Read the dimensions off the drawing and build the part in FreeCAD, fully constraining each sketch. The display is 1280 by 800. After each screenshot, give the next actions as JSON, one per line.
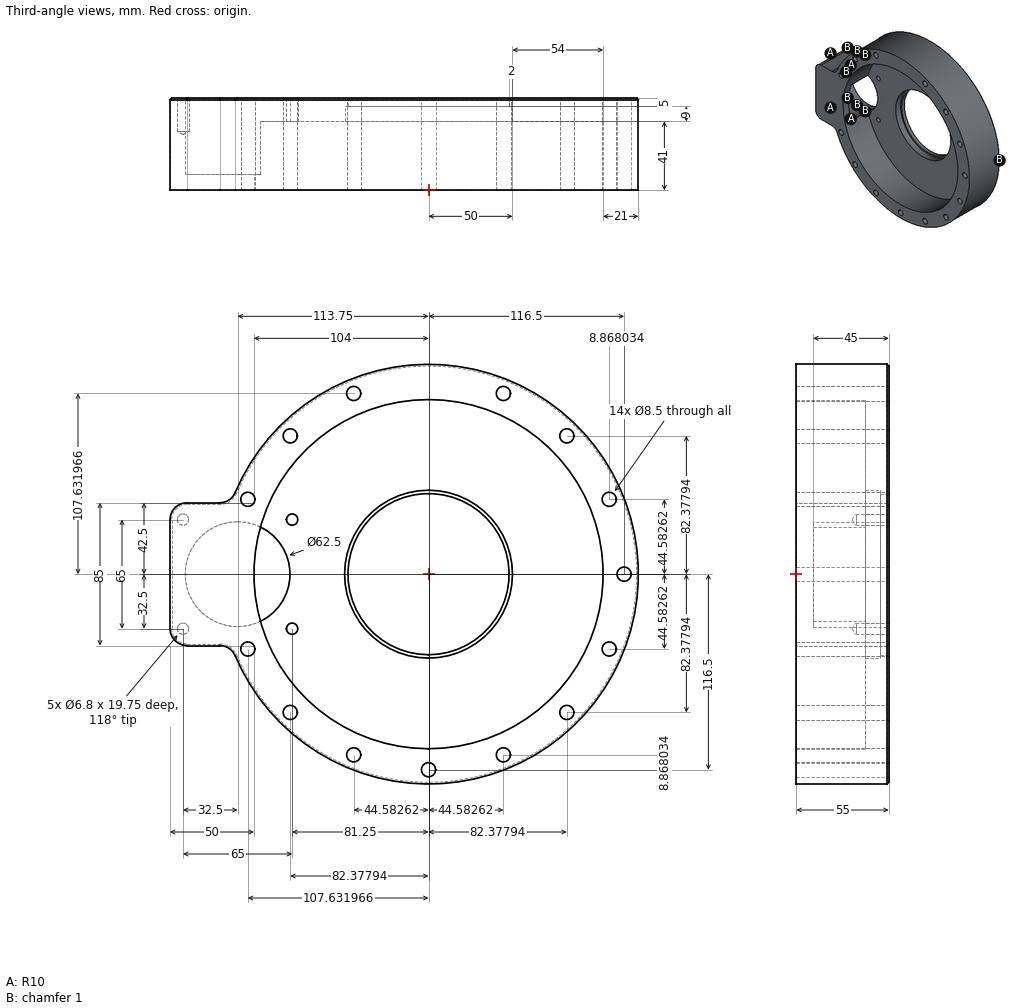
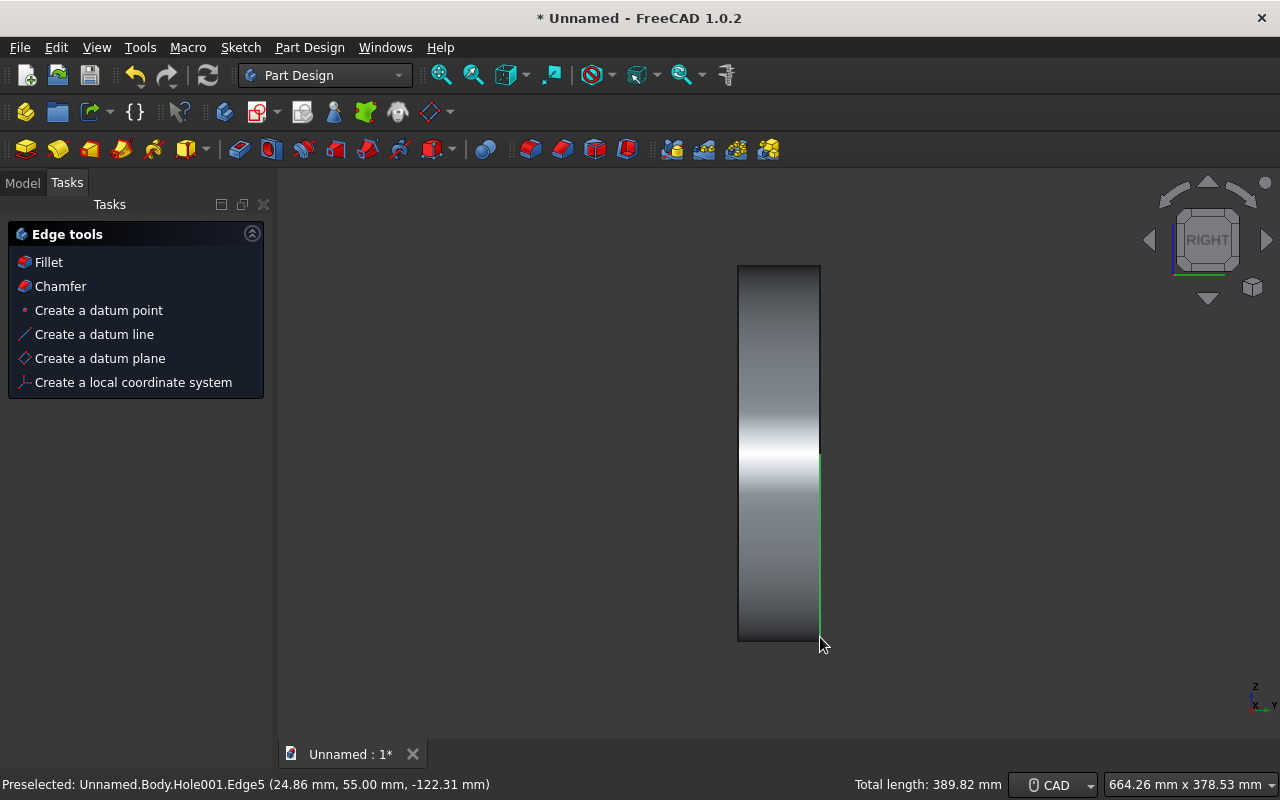
{"action": "key", "text": "5"}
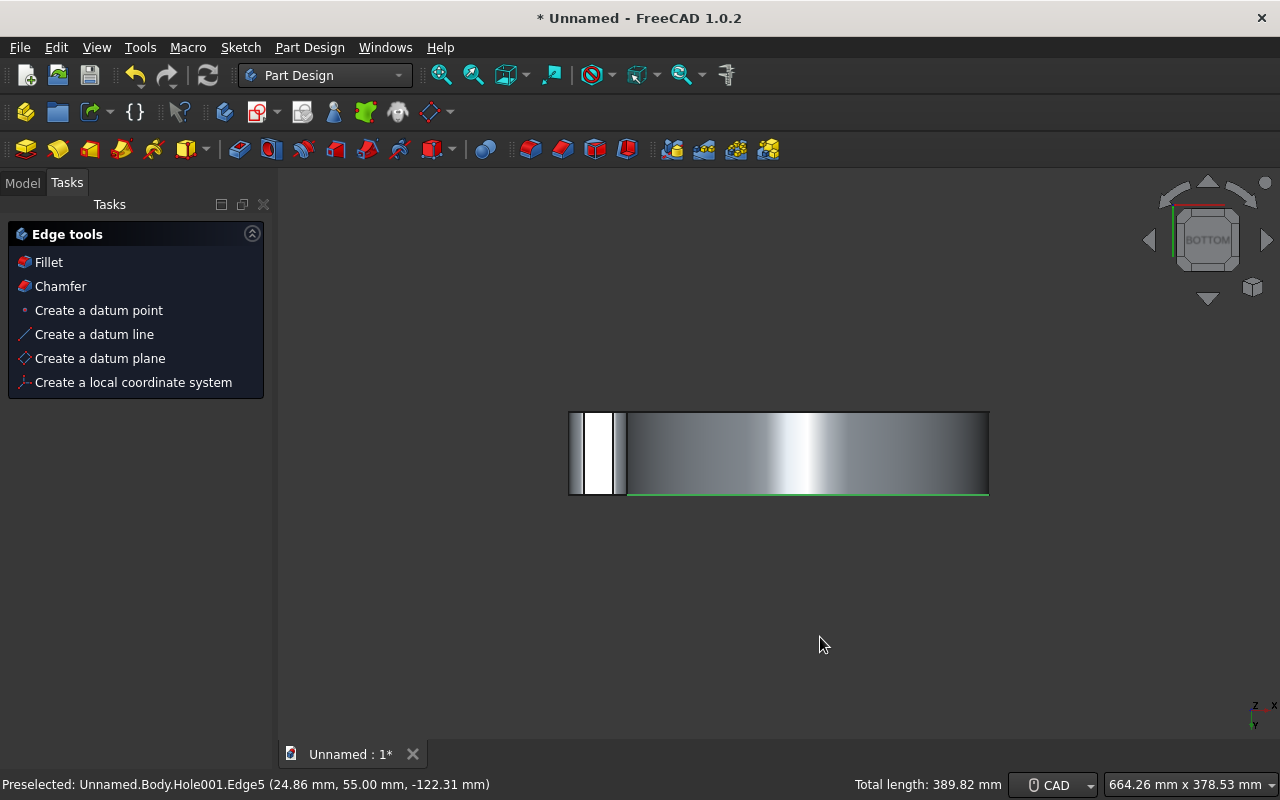
{"action": "left_click", "coordinate": [442, 76]}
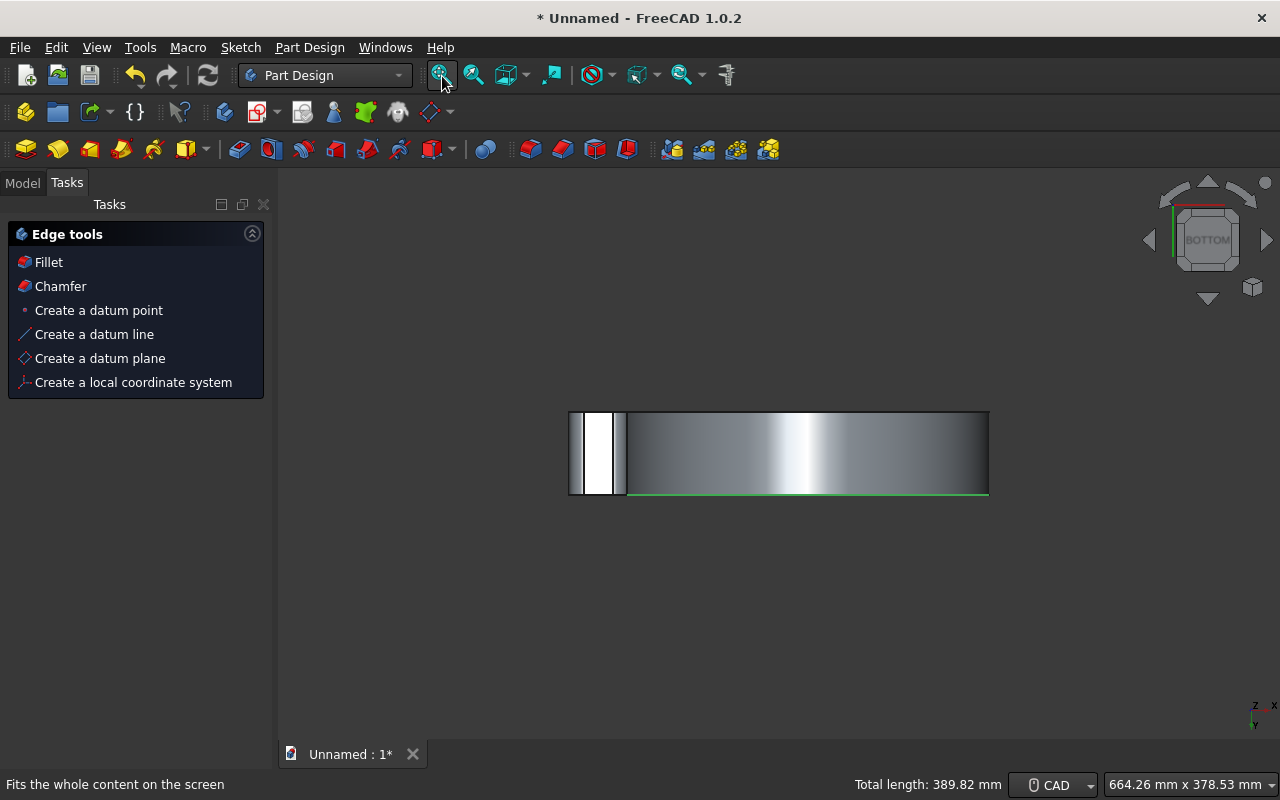
{"action": "left_click", "coordinate": [598, 494], "text": "ctrl"}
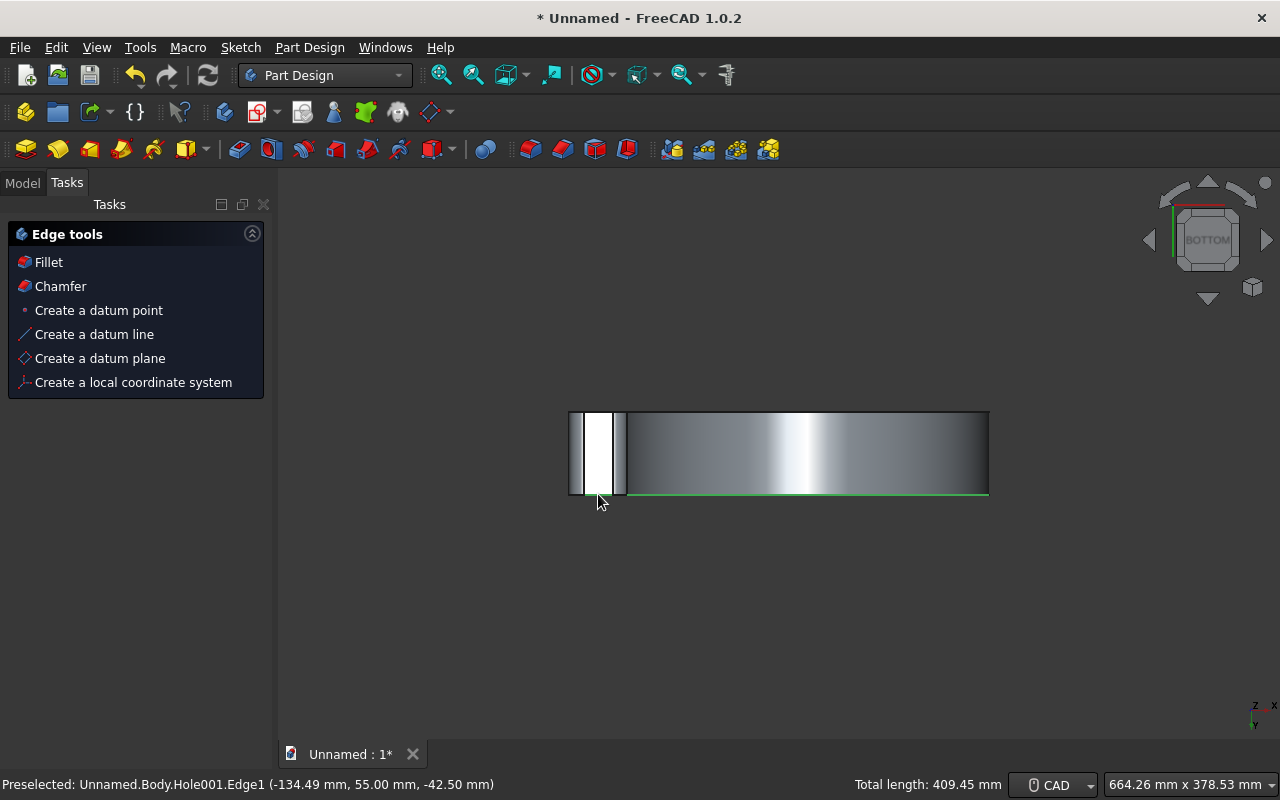
{"action": "left_click", "coordinate": [573, 494], "text": "ctrl"}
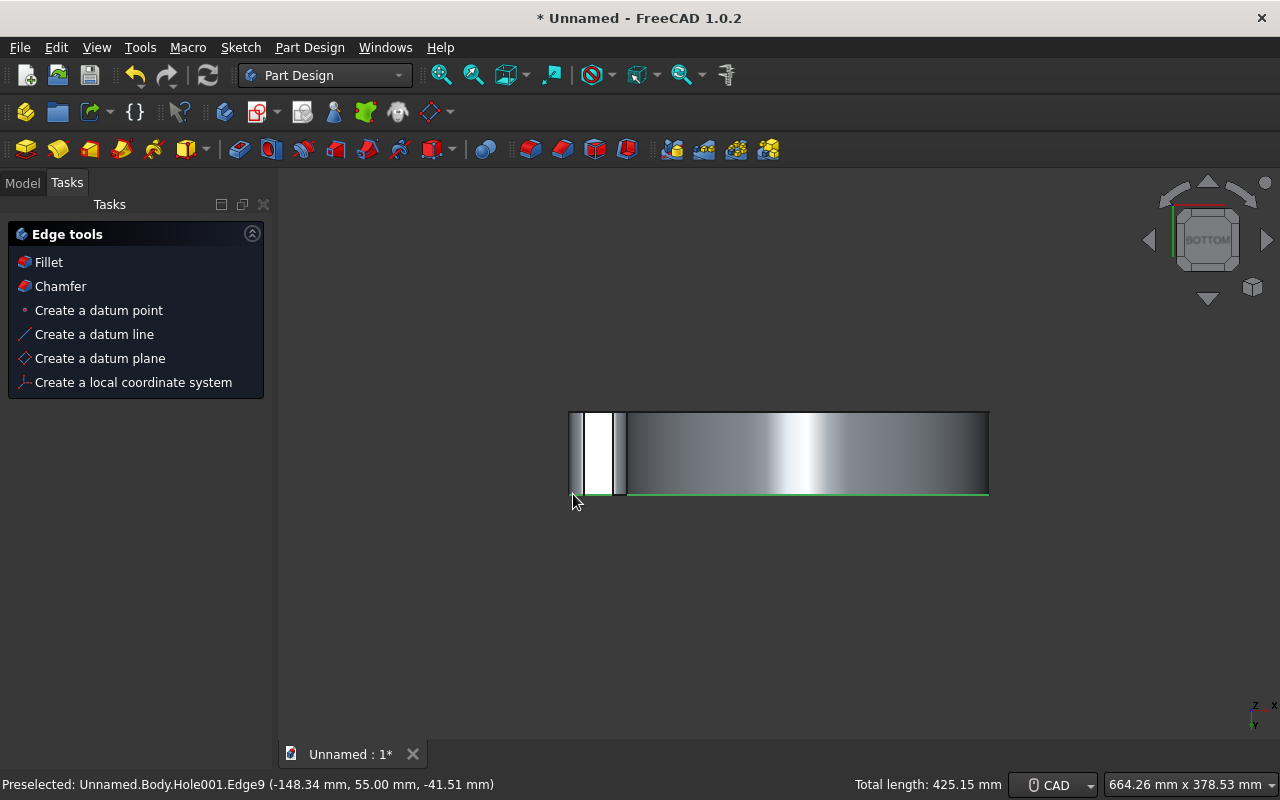
{"action": "left_click", "coordinate": [620, 494], "text": "ctrl"}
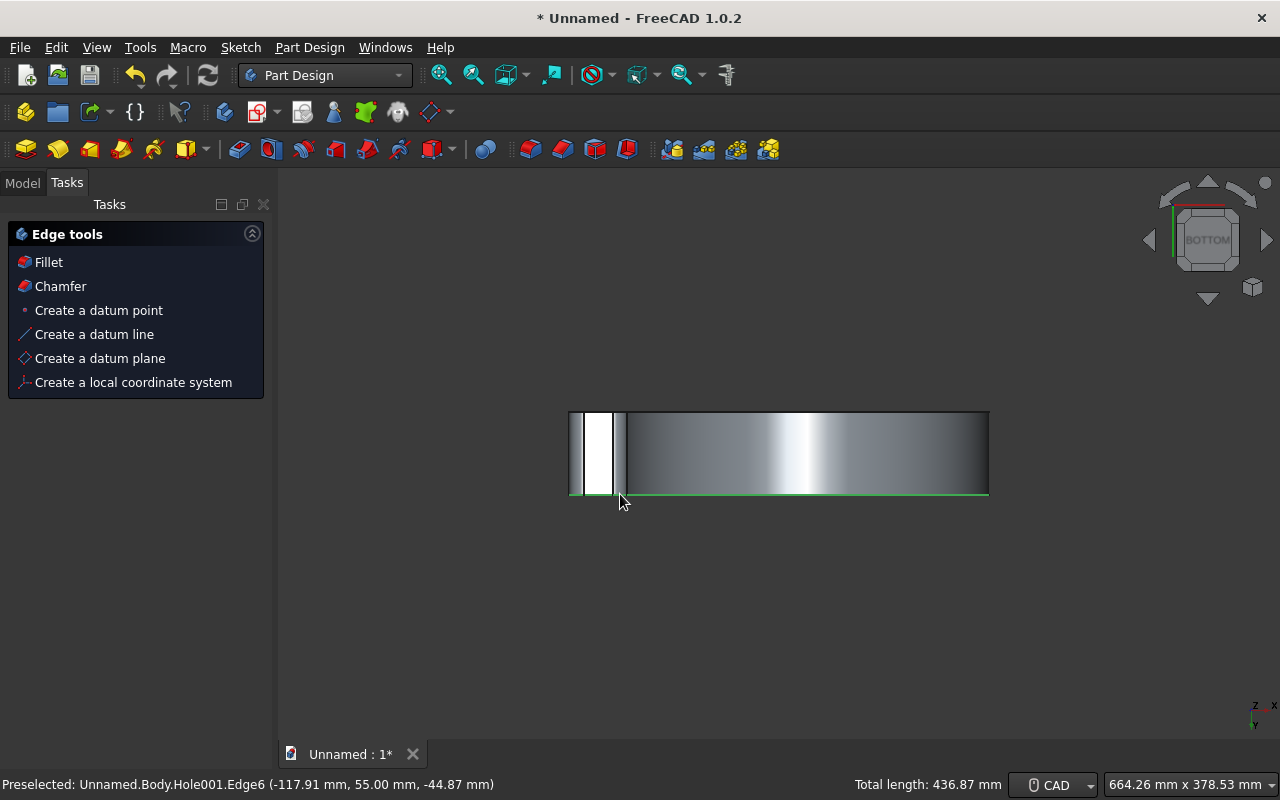
{"action": "key", "text": "4"}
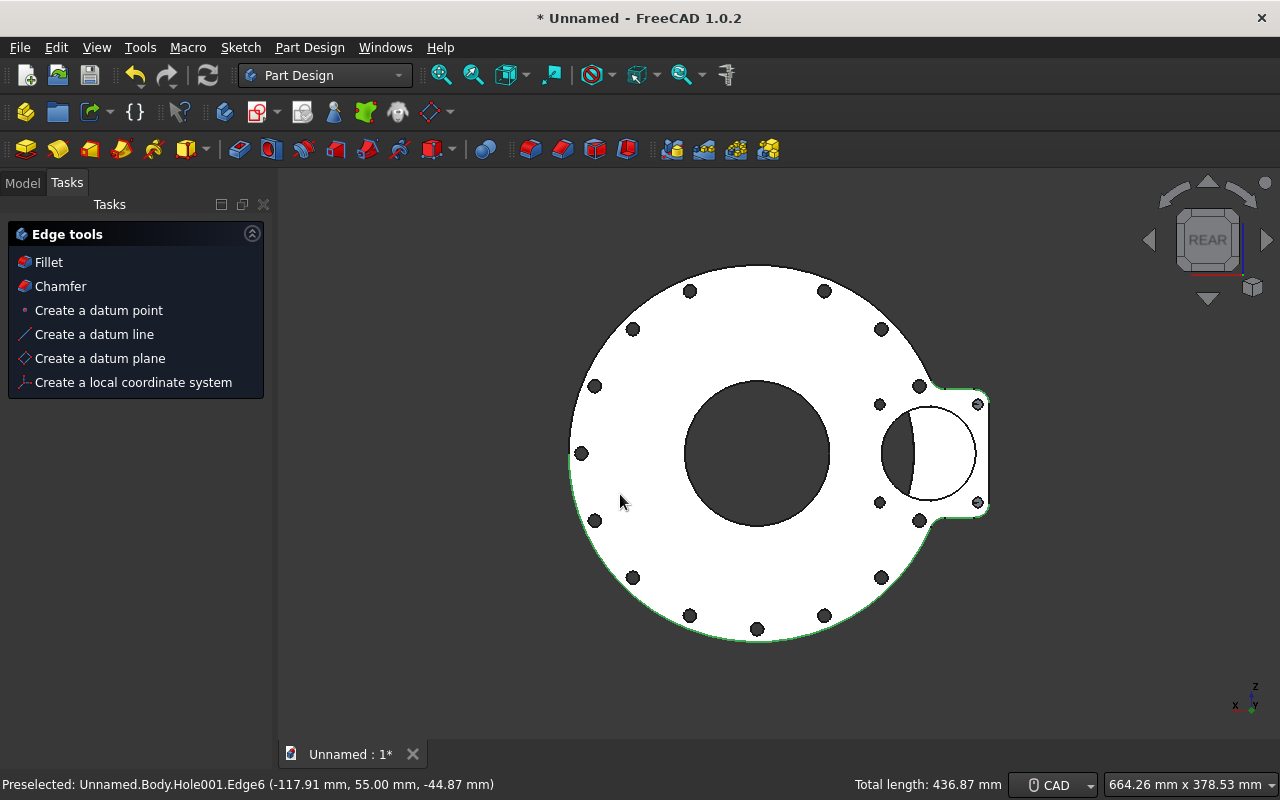
{"action": "left_click", "coordinate": [989, 452], "text": "ctrl"}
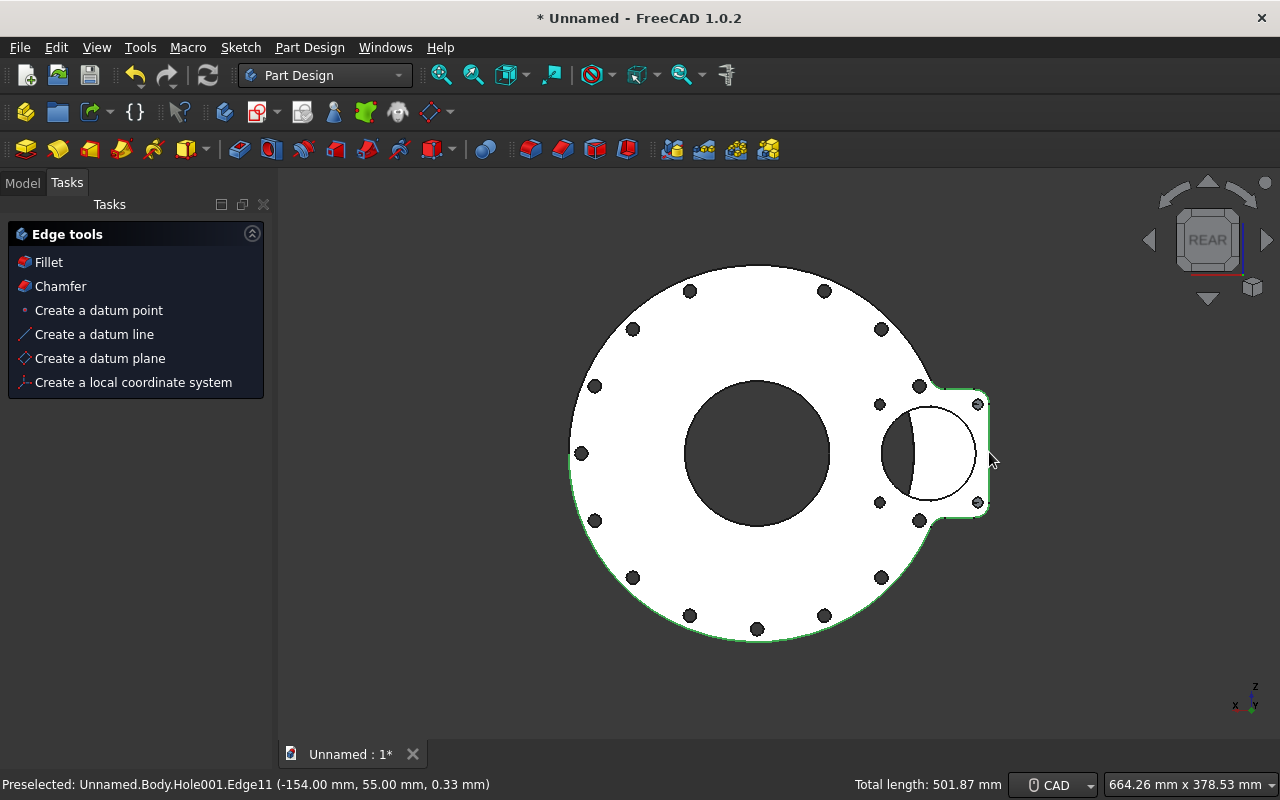
{"action": "left_click", "coordinate": [564, 150]}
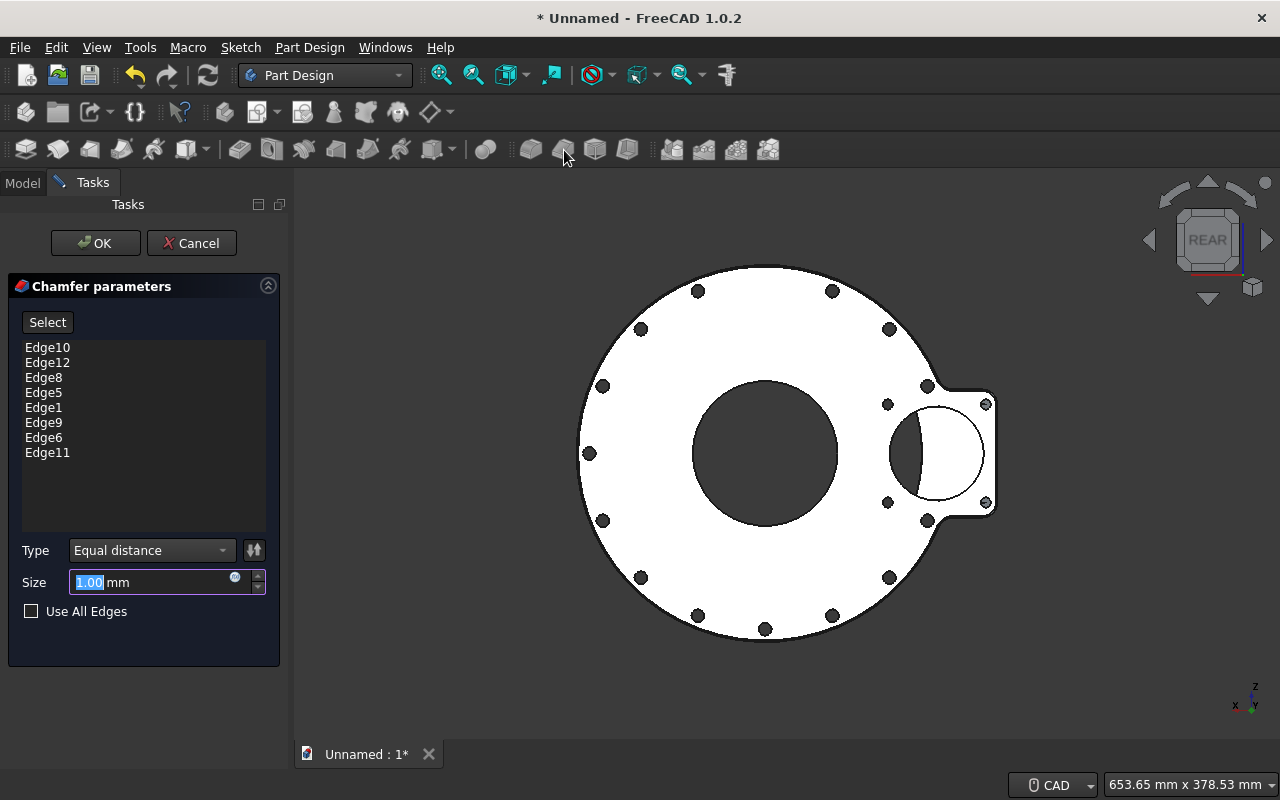
{"action": "type", "text": "1"}
{"action": "key", "text": "Tab"}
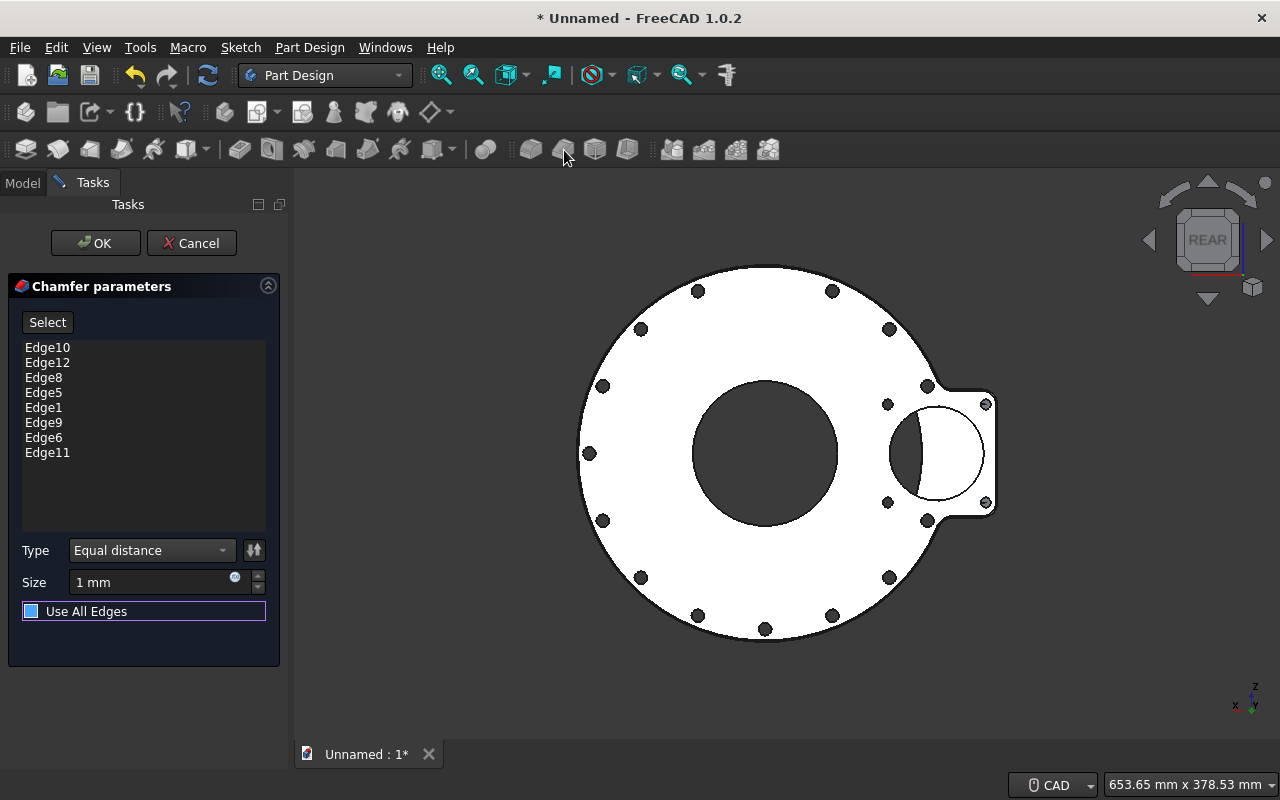
{"action": "left_click", "coordinate": [96, 243]}